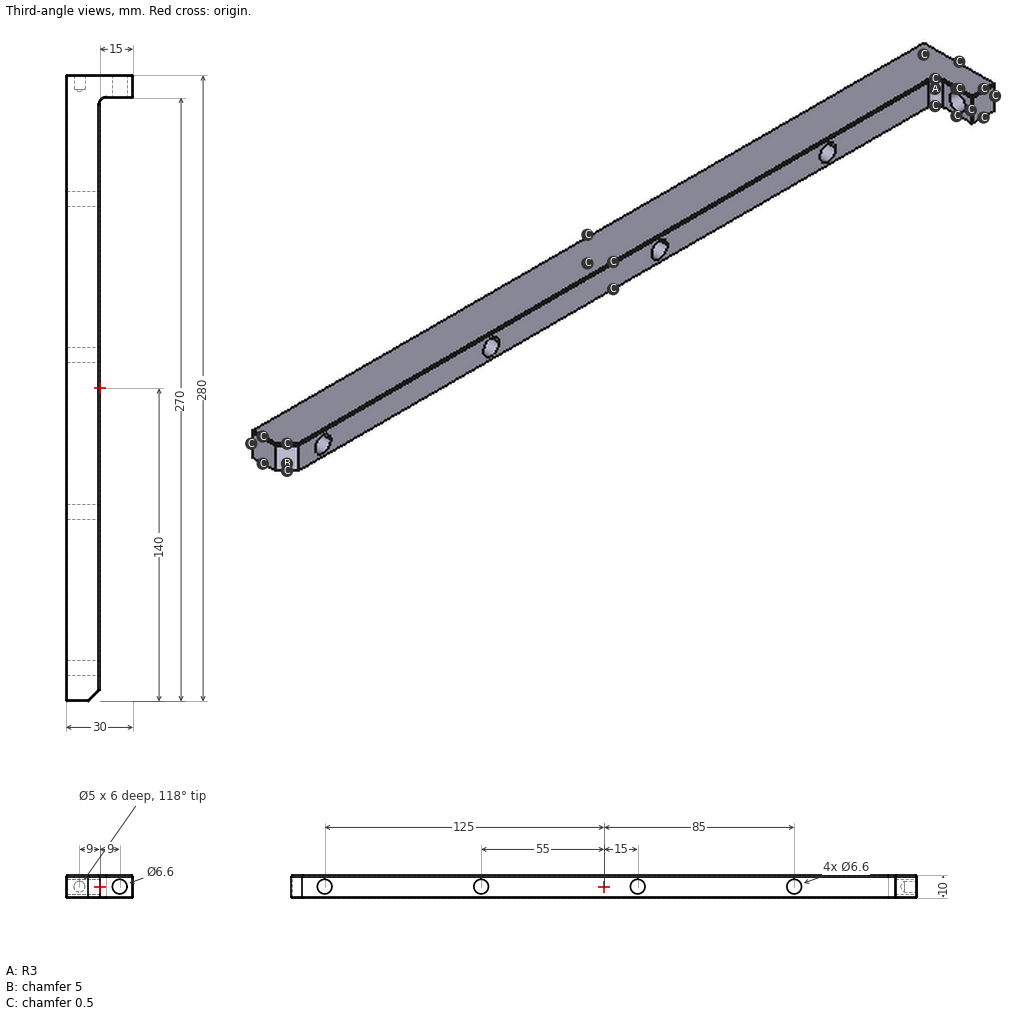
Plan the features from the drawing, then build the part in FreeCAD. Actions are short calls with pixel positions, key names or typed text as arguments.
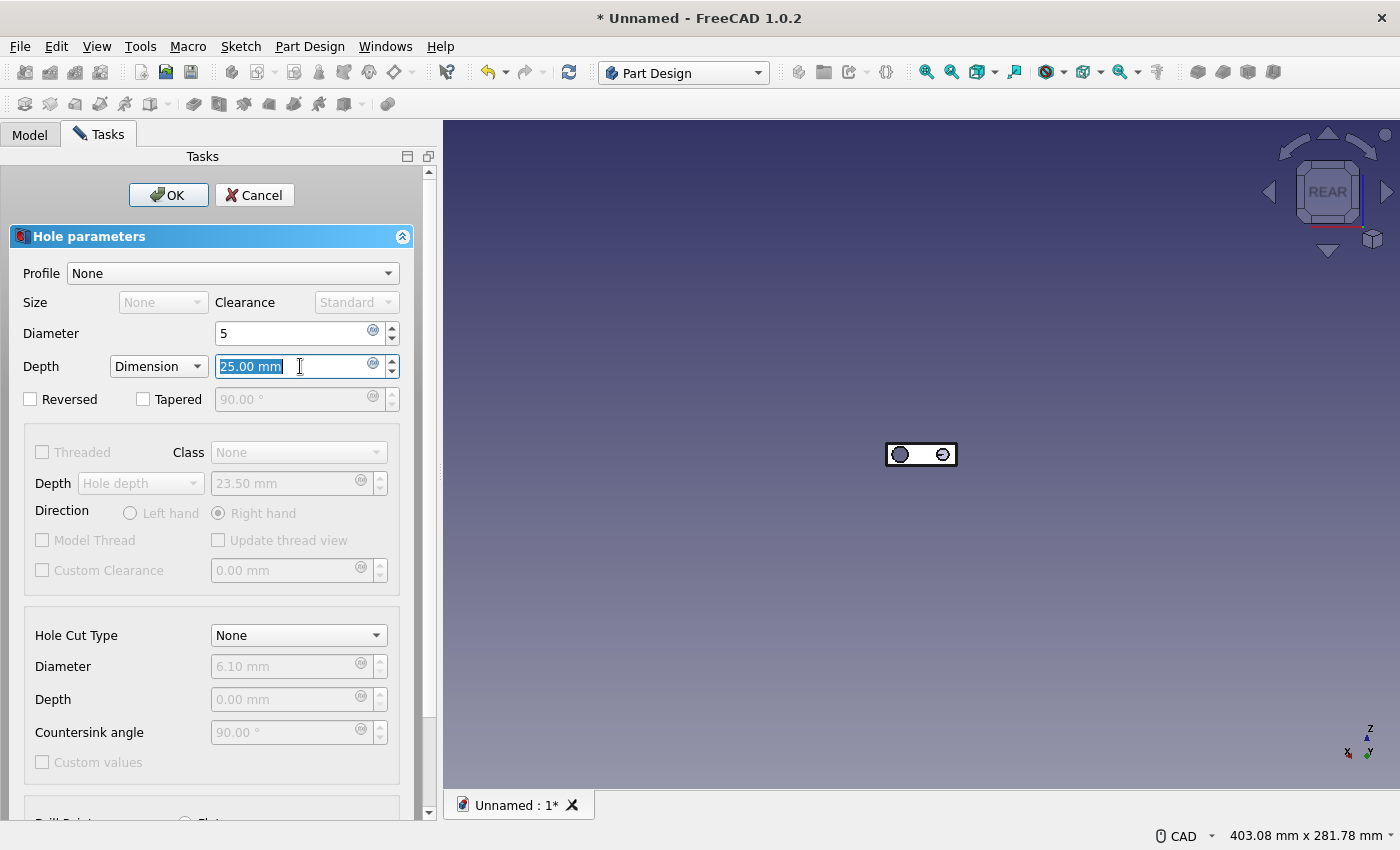
text(6)
key(Tab)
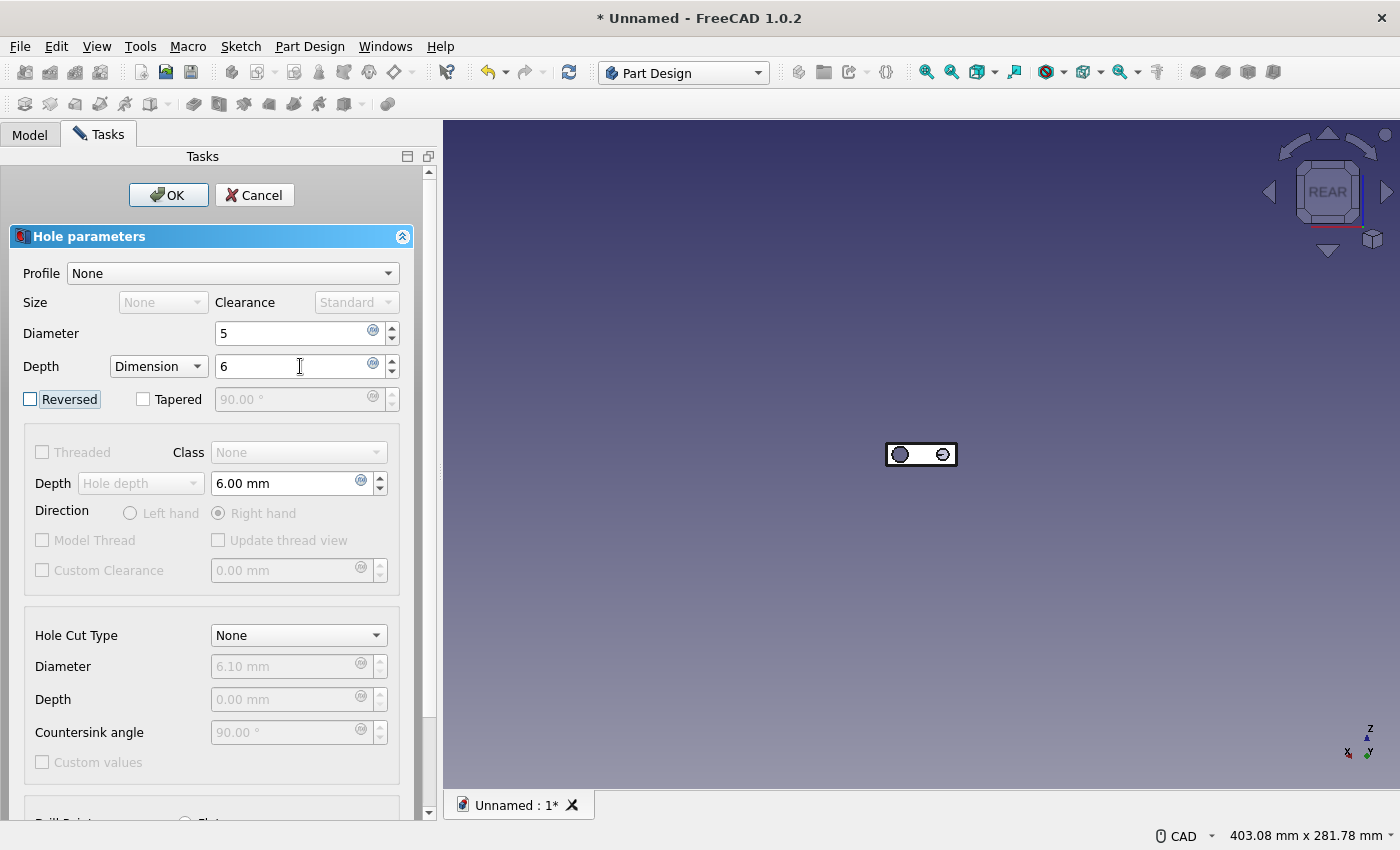
click(169, 195)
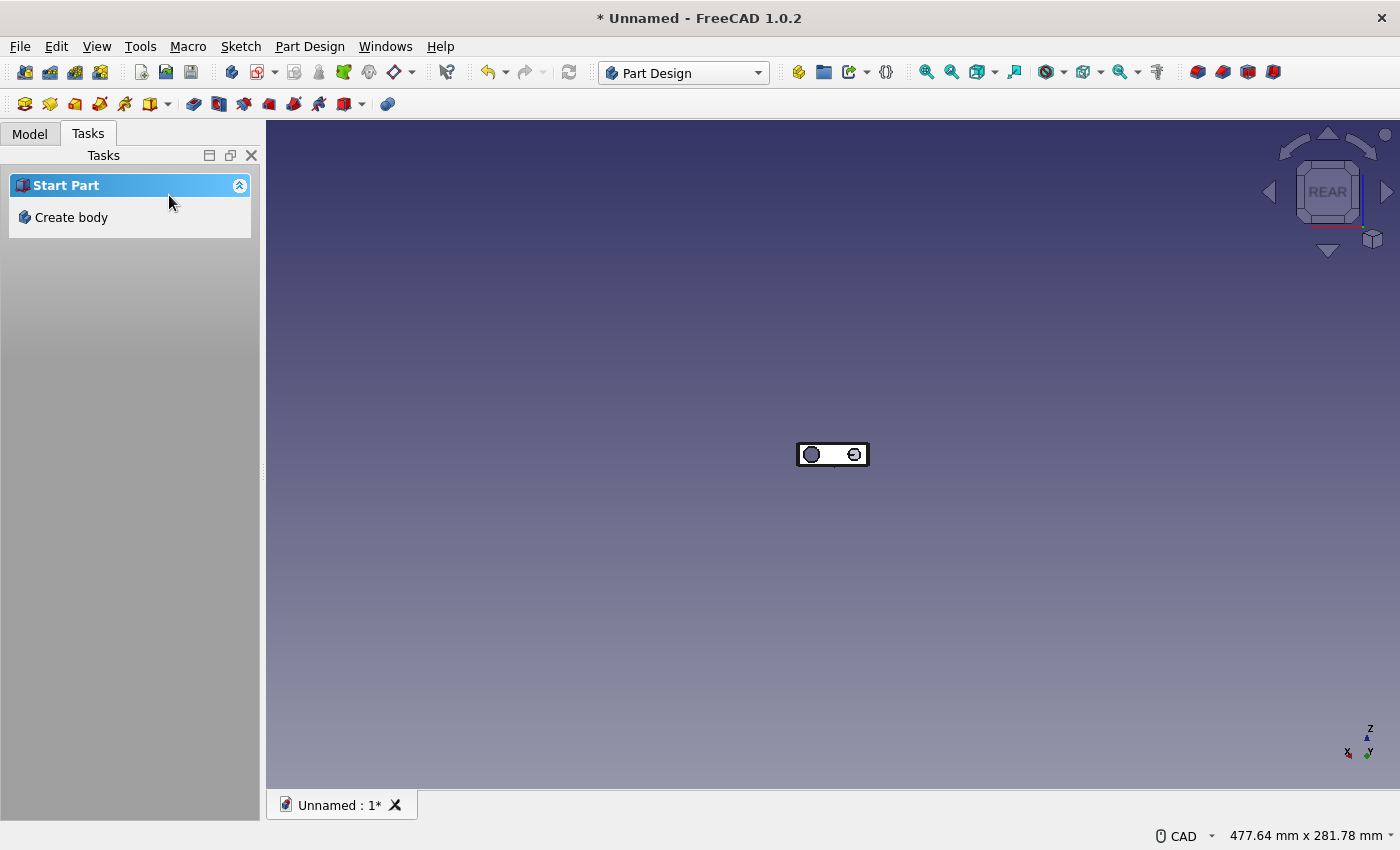
key(0)